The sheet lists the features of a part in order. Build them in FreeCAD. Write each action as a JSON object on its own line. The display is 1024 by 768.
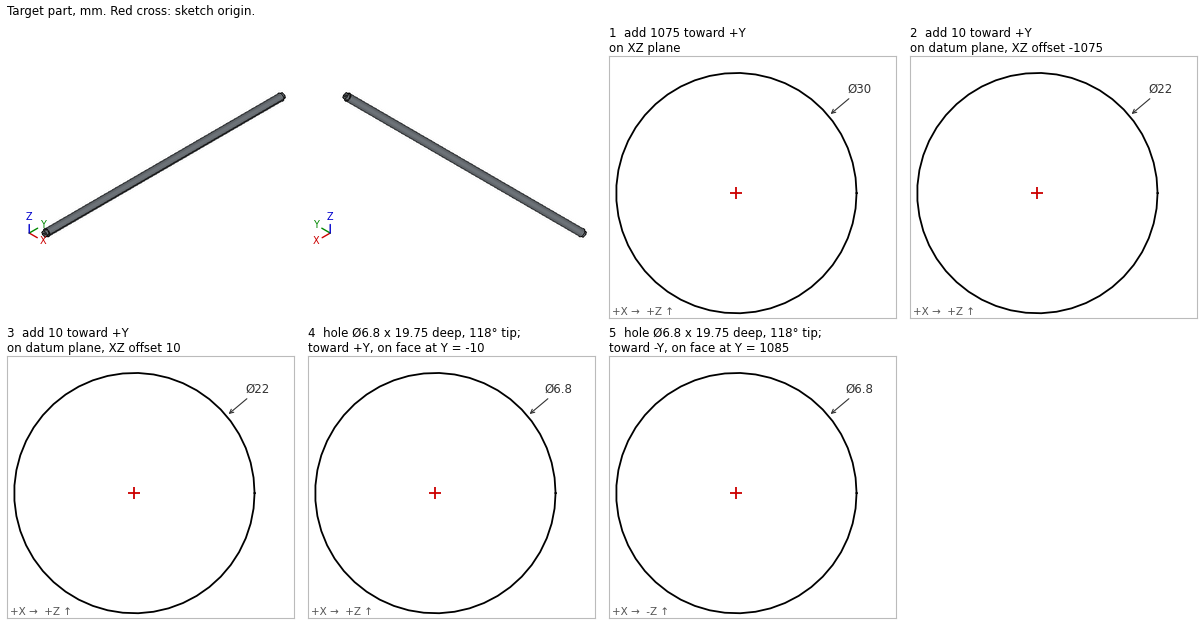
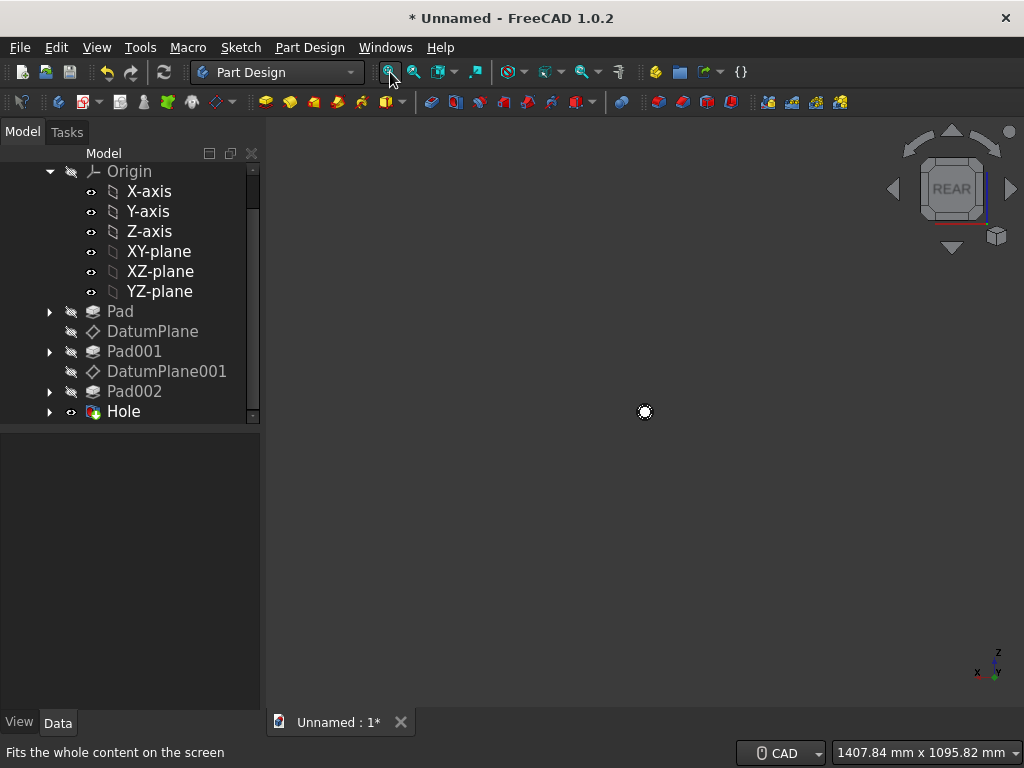
{"action": "left_click", "coordinate": [390, 72]}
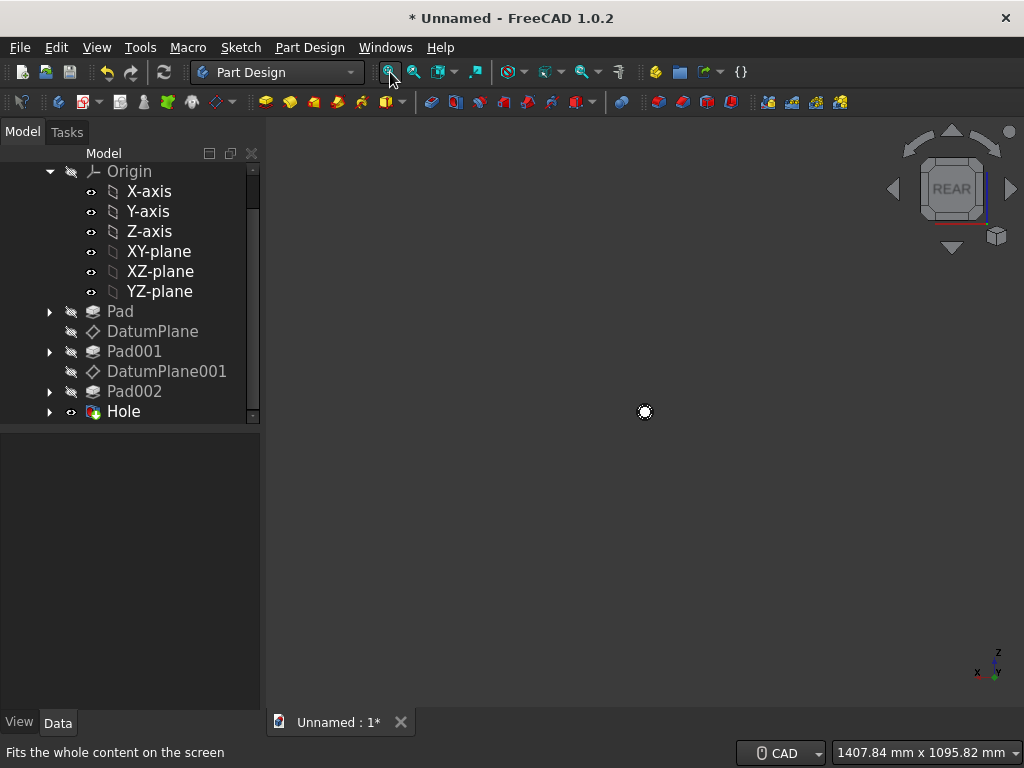
{"action": "scroll", "coordinate": [645, 411], "scroll_direction": "up", "scroll_amount": 4}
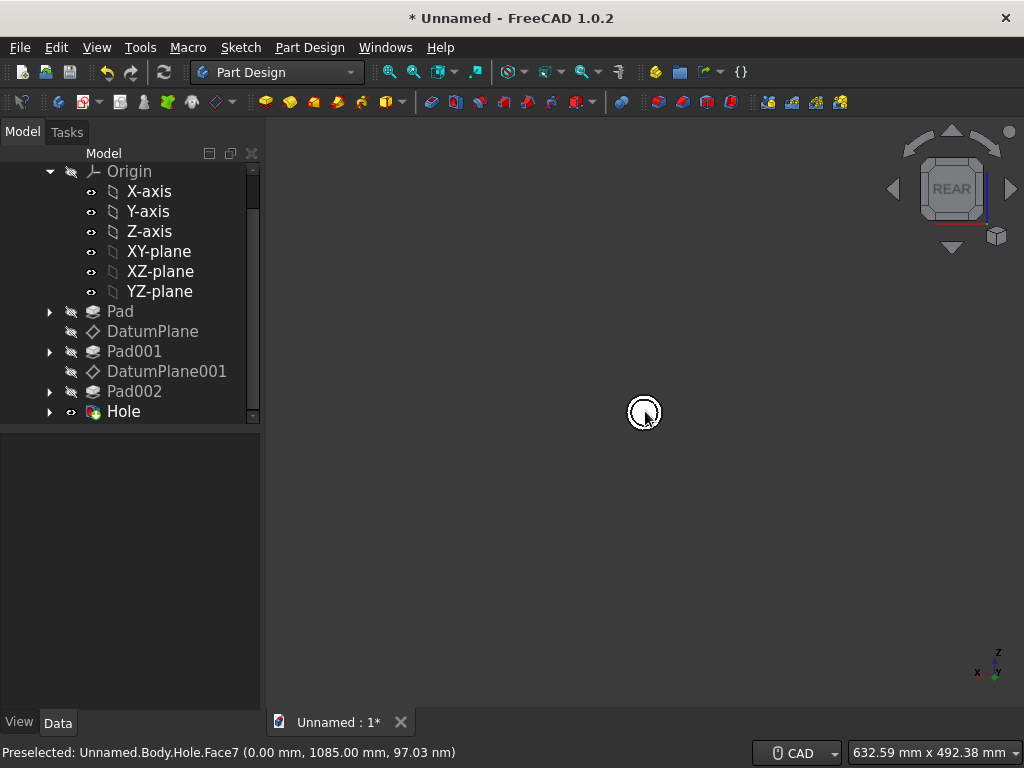
{"action": "left_click", "coordinate": [644, 412]}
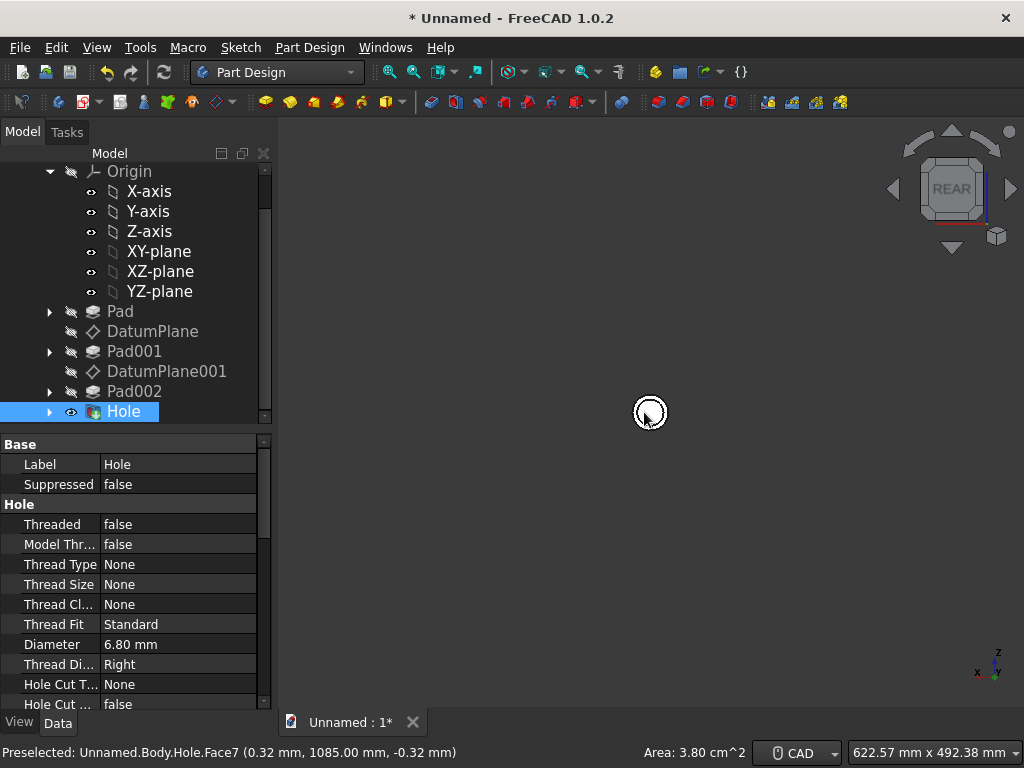
{"action": "left_click", "coordinate": [84, 102]}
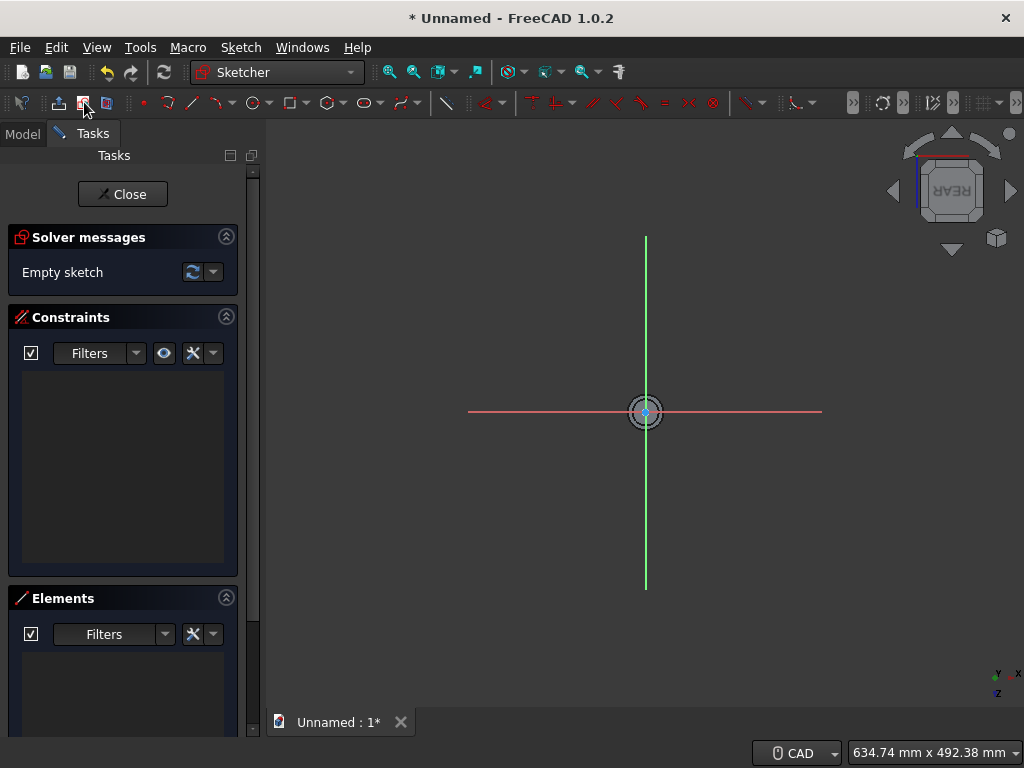
{"action": "scroll", "coordinate": [649, 412], "scroll_direction": "up", "scroll_amount": 15}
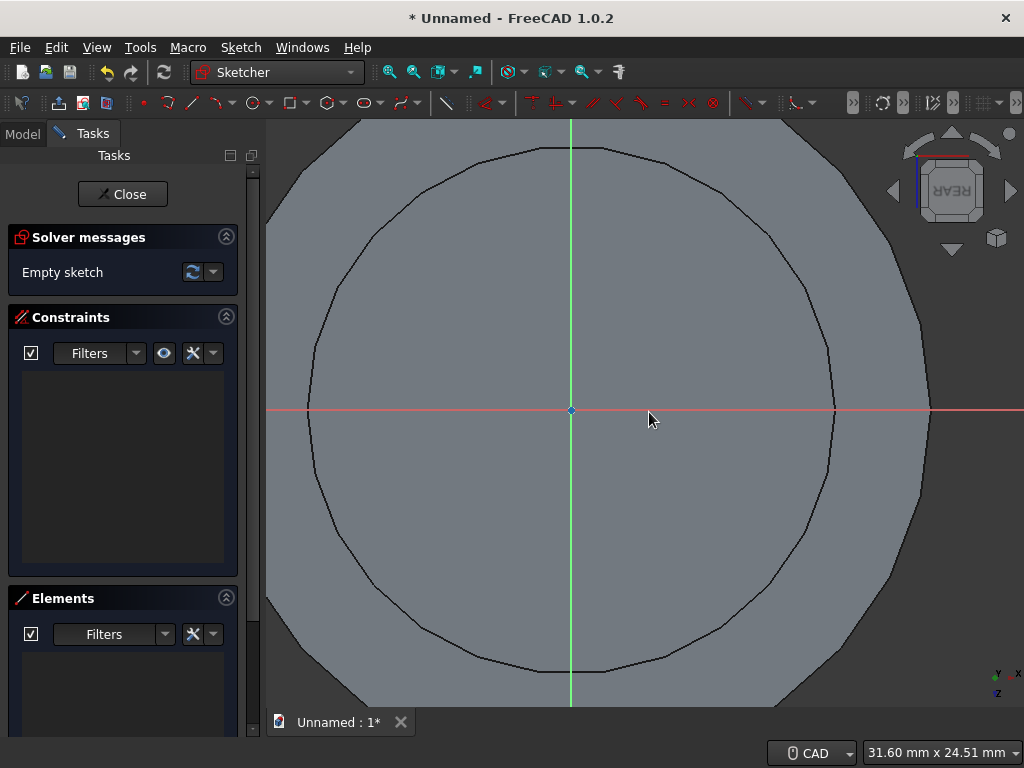
{"action": "scroll", "coordinate": [567, 408], "scroll_direction": "up", "scroll_amount": 4}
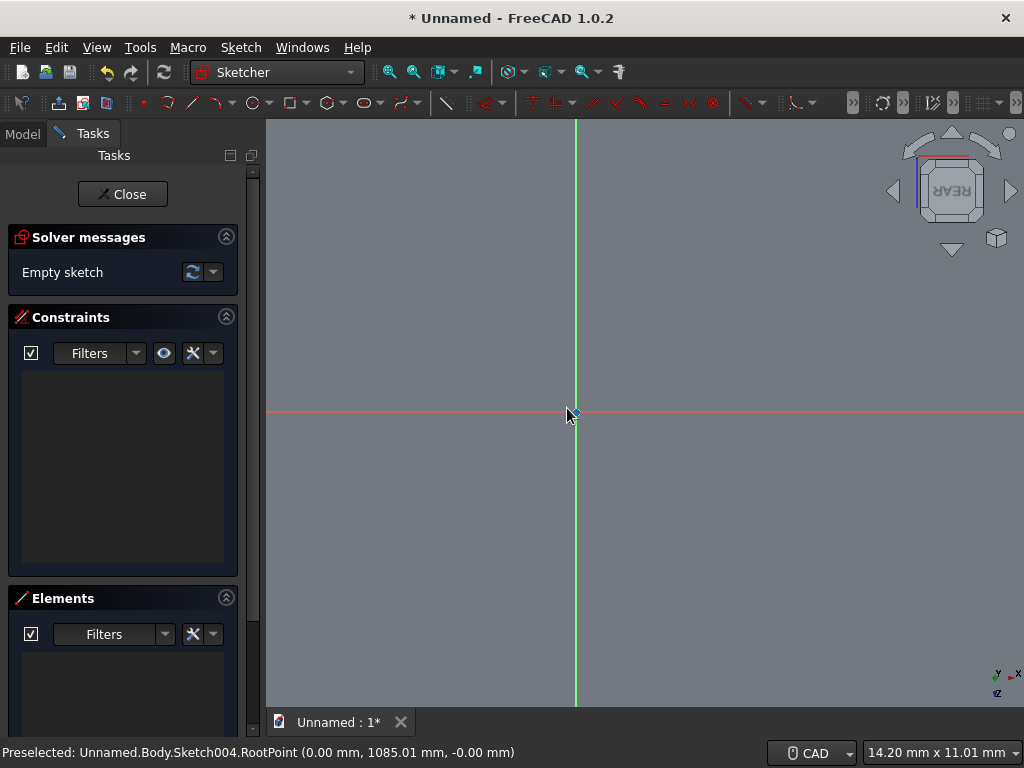
{"action": "left_click", "coordinate": [254, 104]}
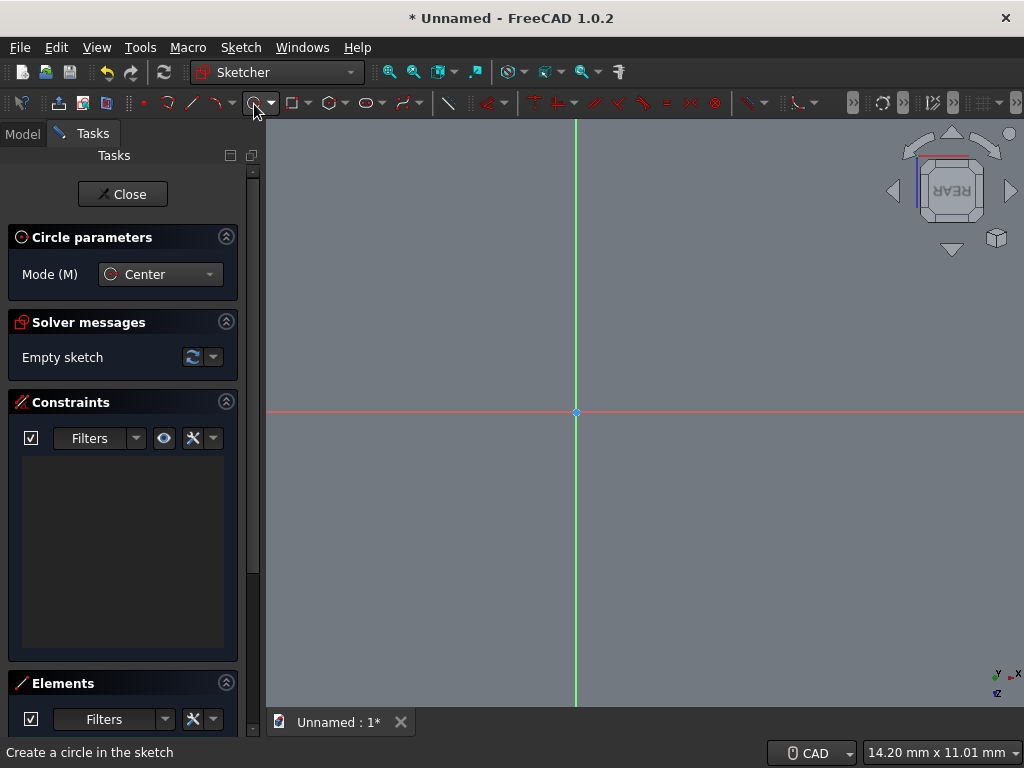
{"action": "left_click", "coordinate": [576, 412]}
{"action": "mouse_move", "coordinate": [704, 284]}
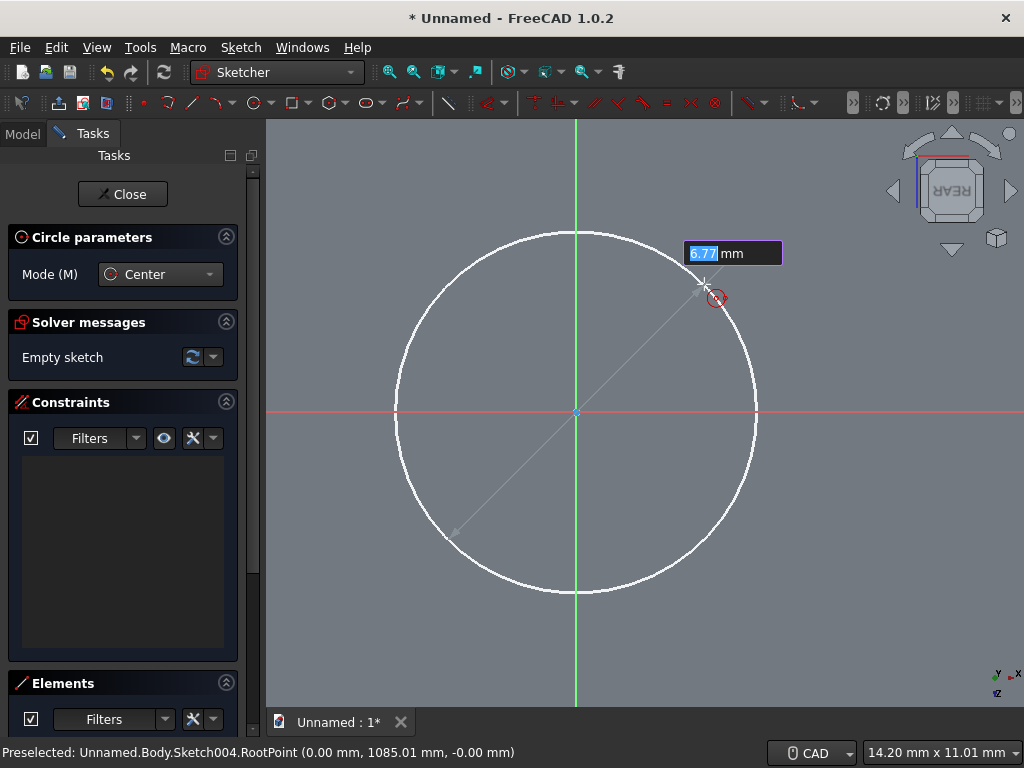
{"action": "type", "text": "6.8"}
{"action": "key", "text": "Return"}
{"action": "key", "text": "Escape"}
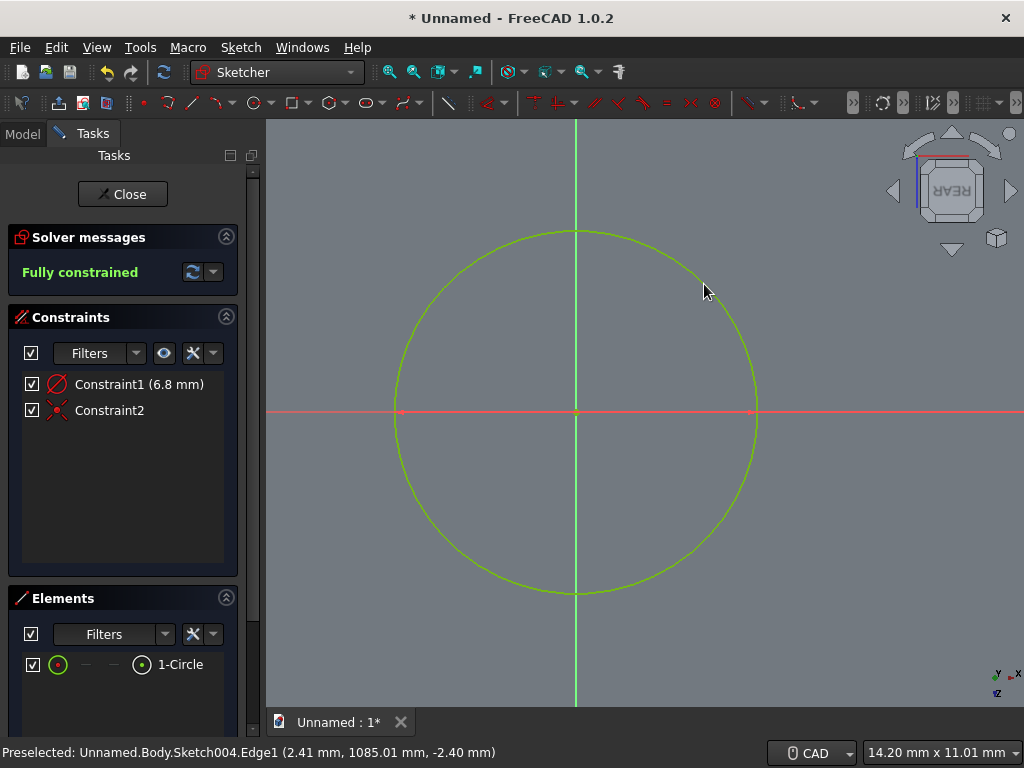
{"action": "left_click", "coordinate": [123, 194]}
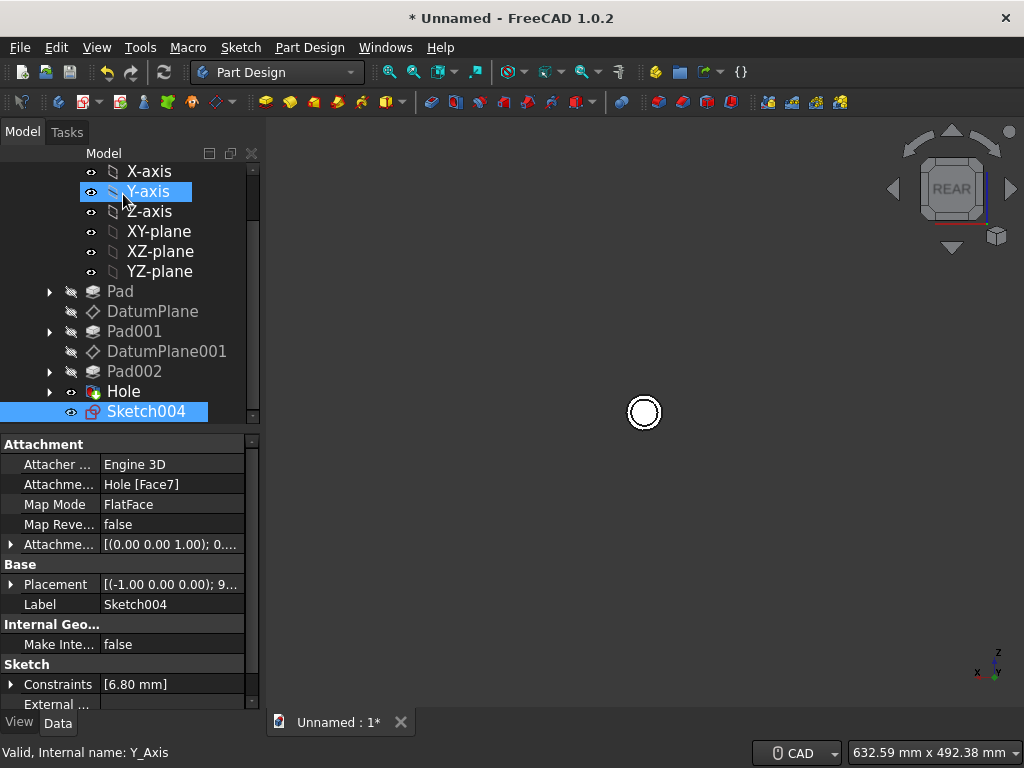
{"action": "left_click", "coordinate": [456, 102]}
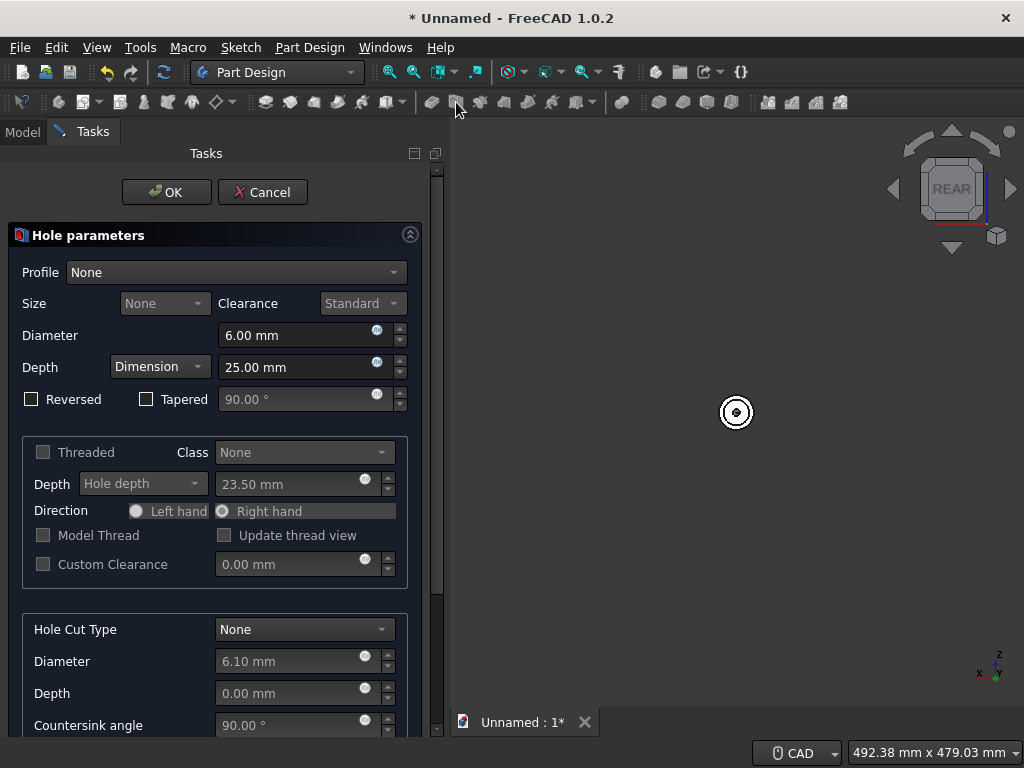
{"action": "triple_click", "coordinate": [305, 335]}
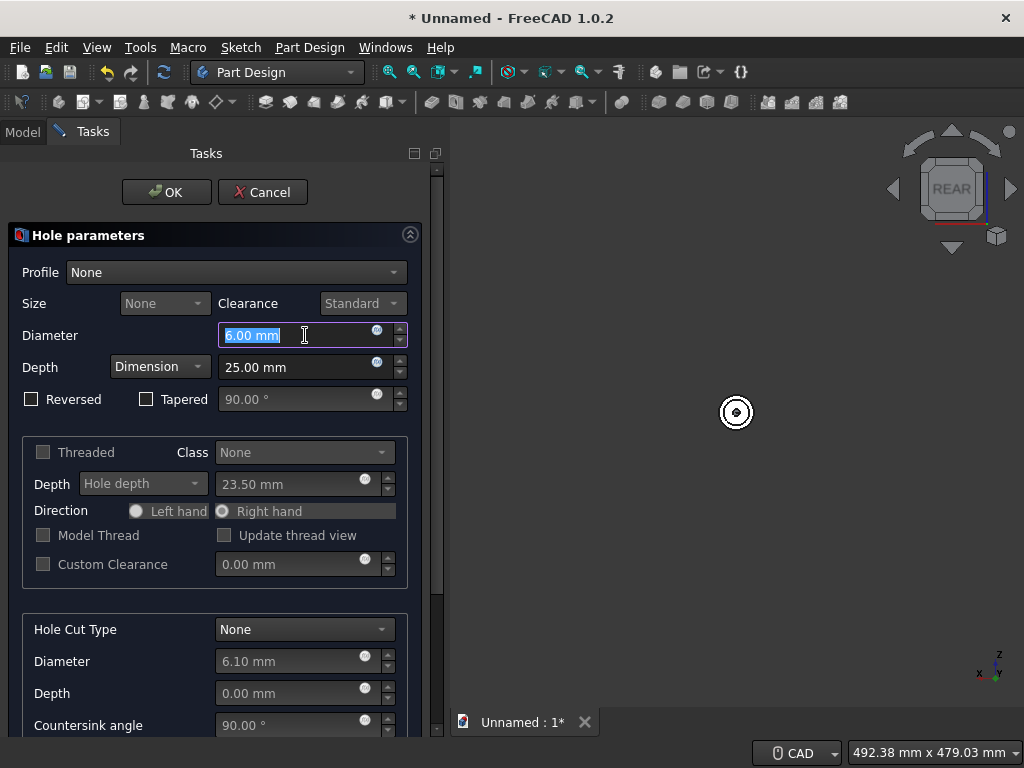
{"action": "type", "text": "6.8"}
{"action": "key", "text": "Tab"}